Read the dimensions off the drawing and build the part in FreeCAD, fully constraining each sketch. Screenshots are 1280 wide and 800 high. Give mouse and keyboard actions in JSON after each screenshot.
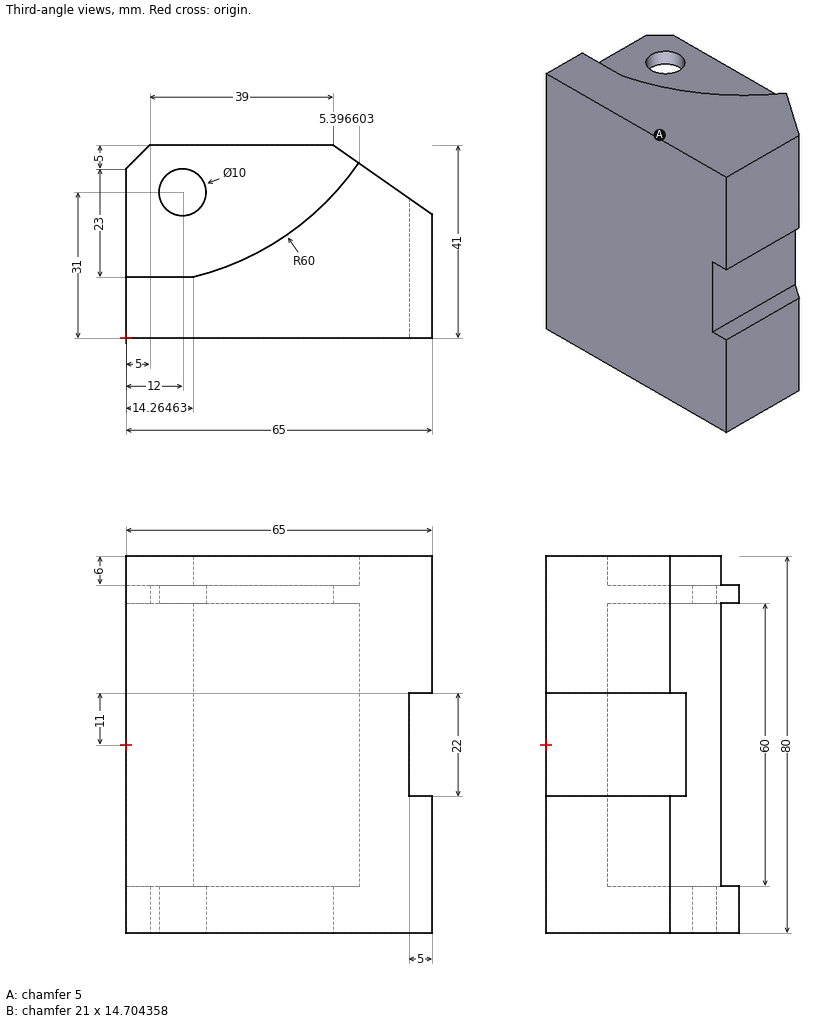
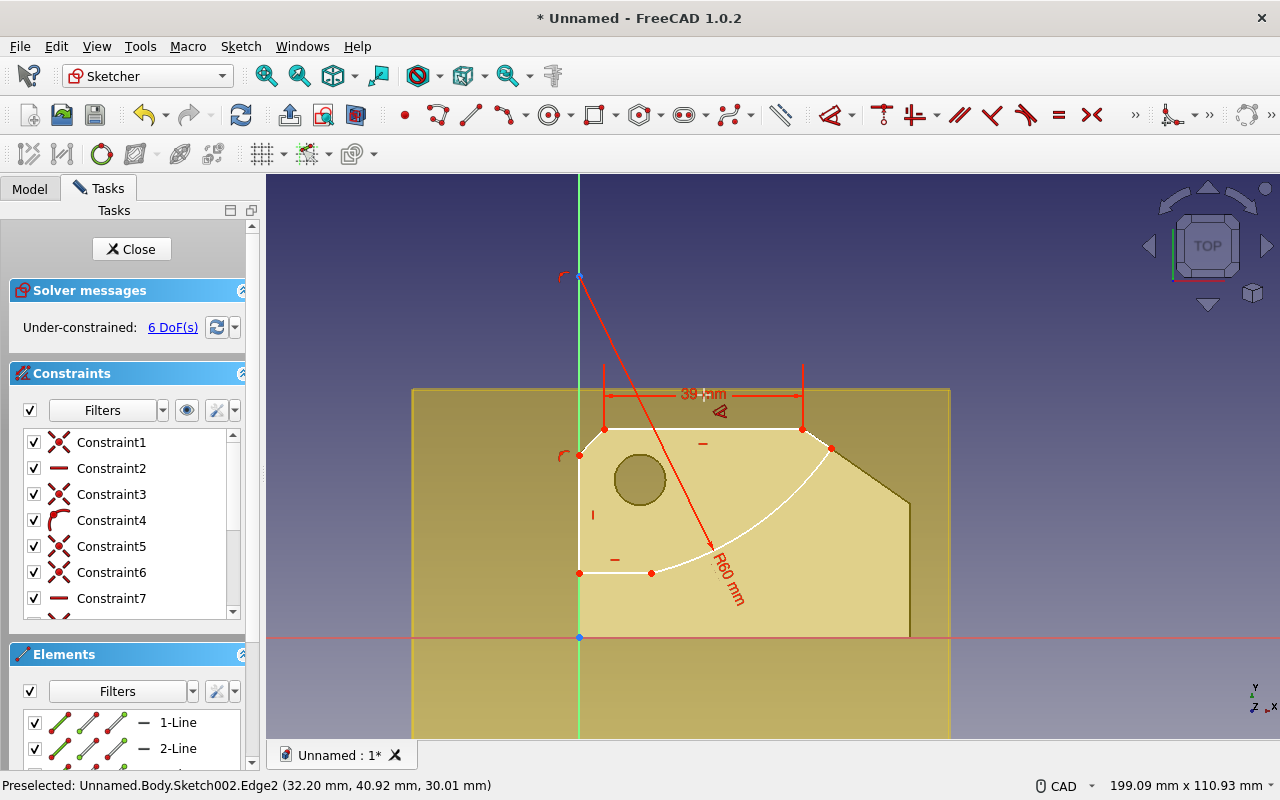
{"action": "left_click", "coordinate": [579, 491]}
{"action": "left_click", "coordinate": [545, 514]}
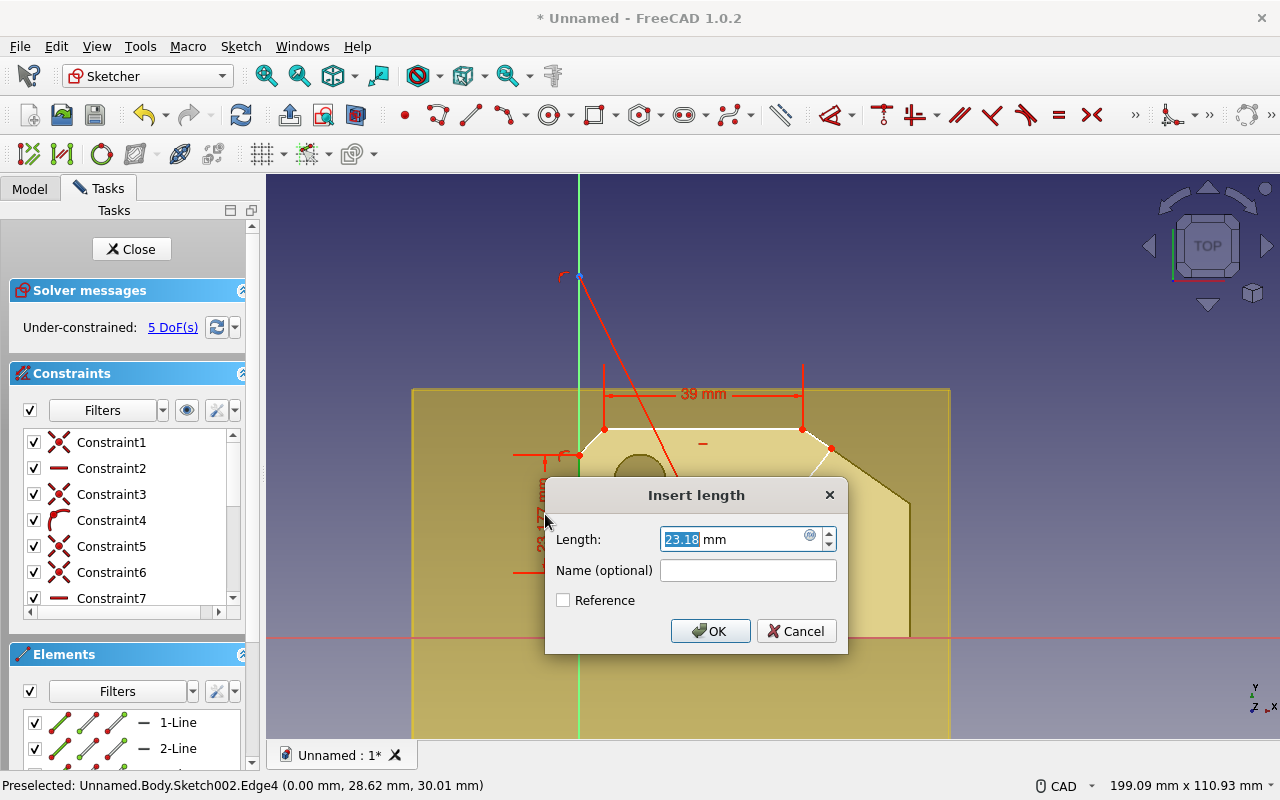
{"action": "type", "text": "23"}
{"action": "key", "text": "Return"}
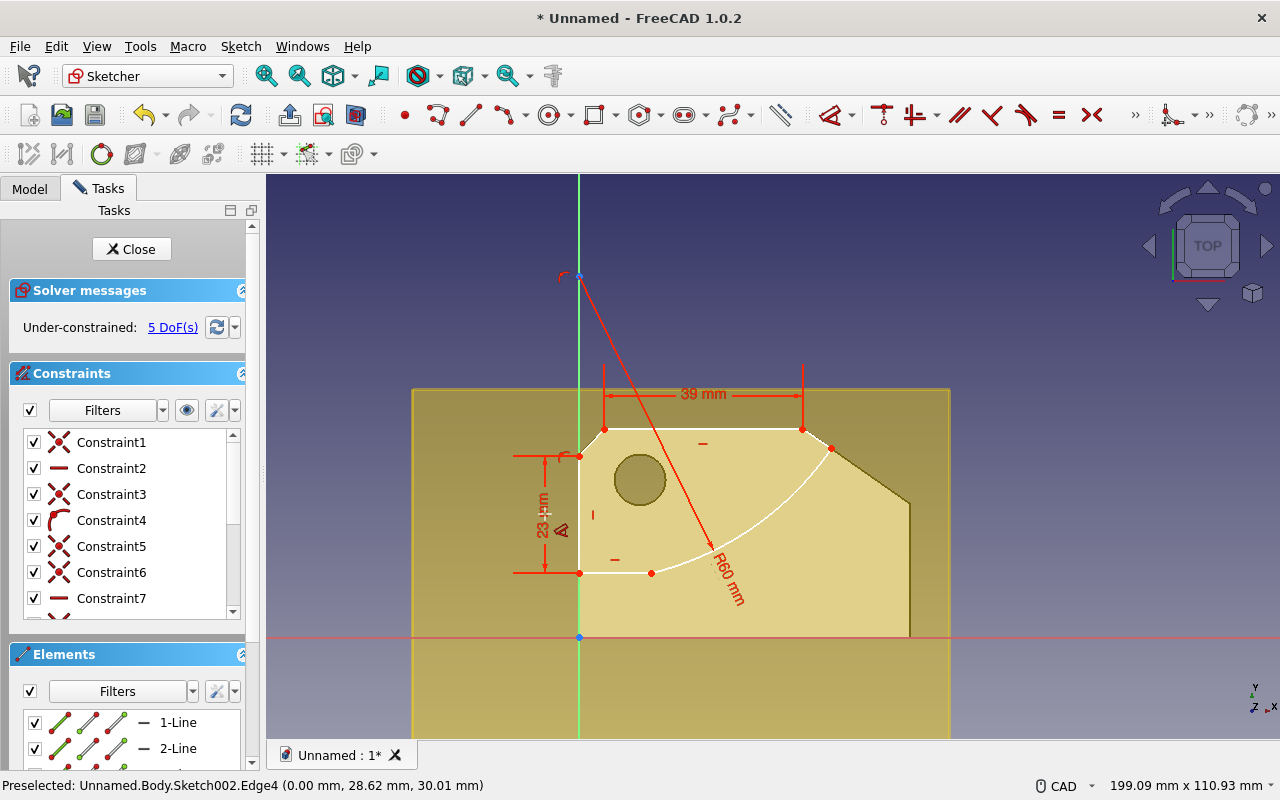
{"action": "scroll", "coordinate": [604, 429], "scroll_direction": "up", "scroll_amount": 3}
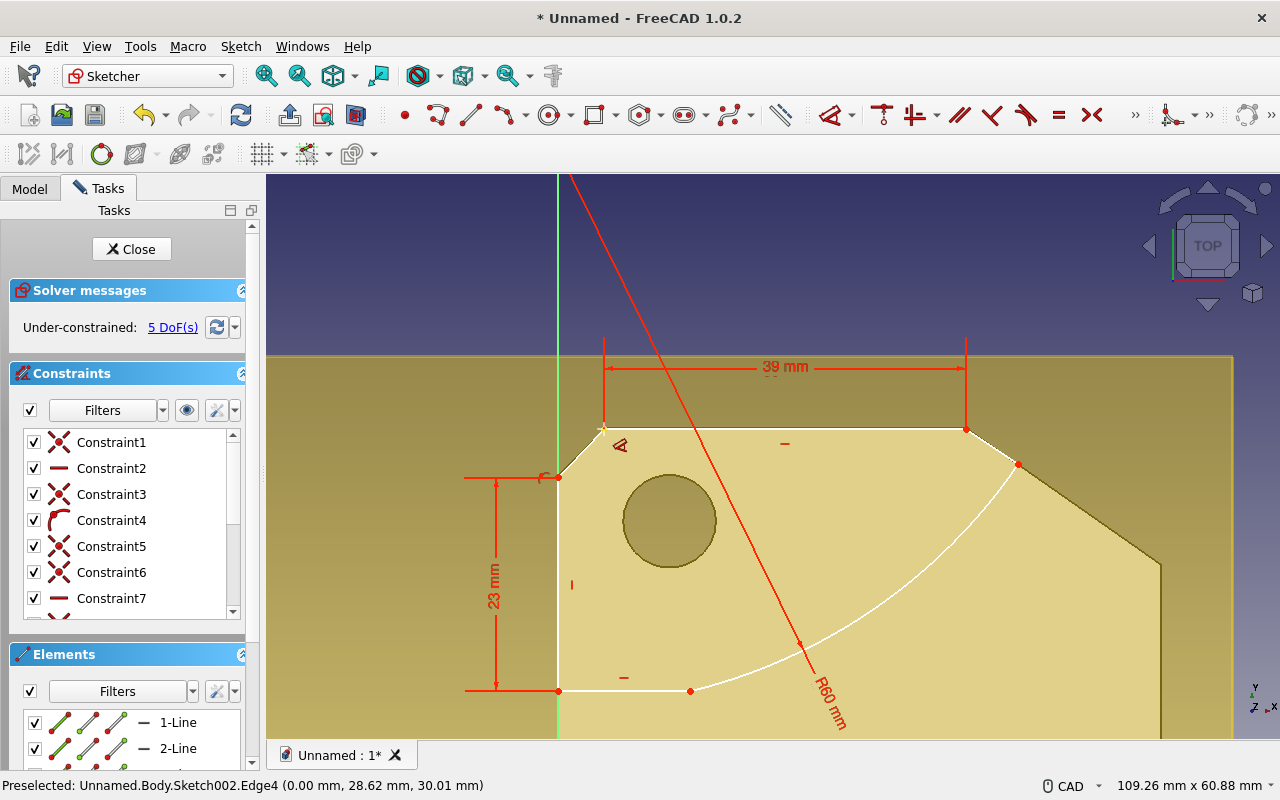
{"action": "left_click", "coordinate": [604, 429]}
{"action": "left_click", "coordinate": [581, 395]}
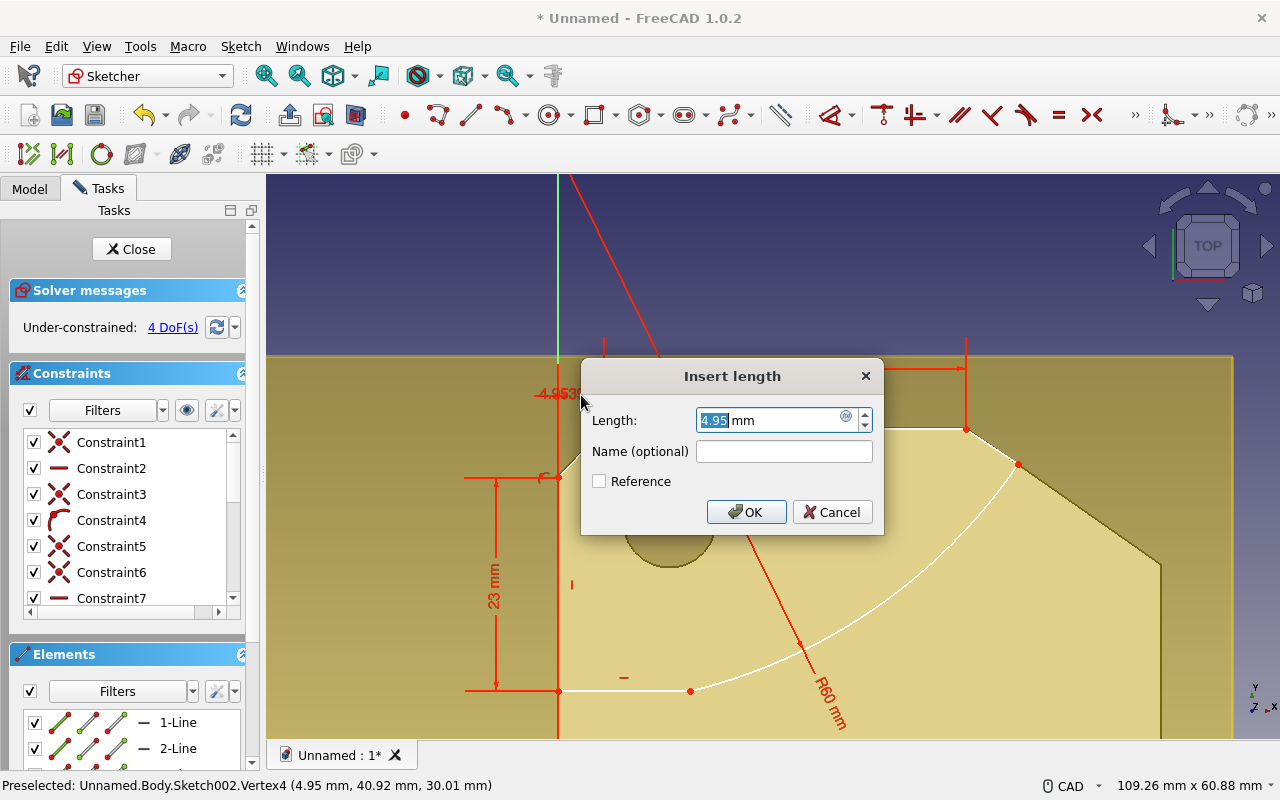
{"action": "type", "text": "5"}
{"action": "key", "text": "Return"}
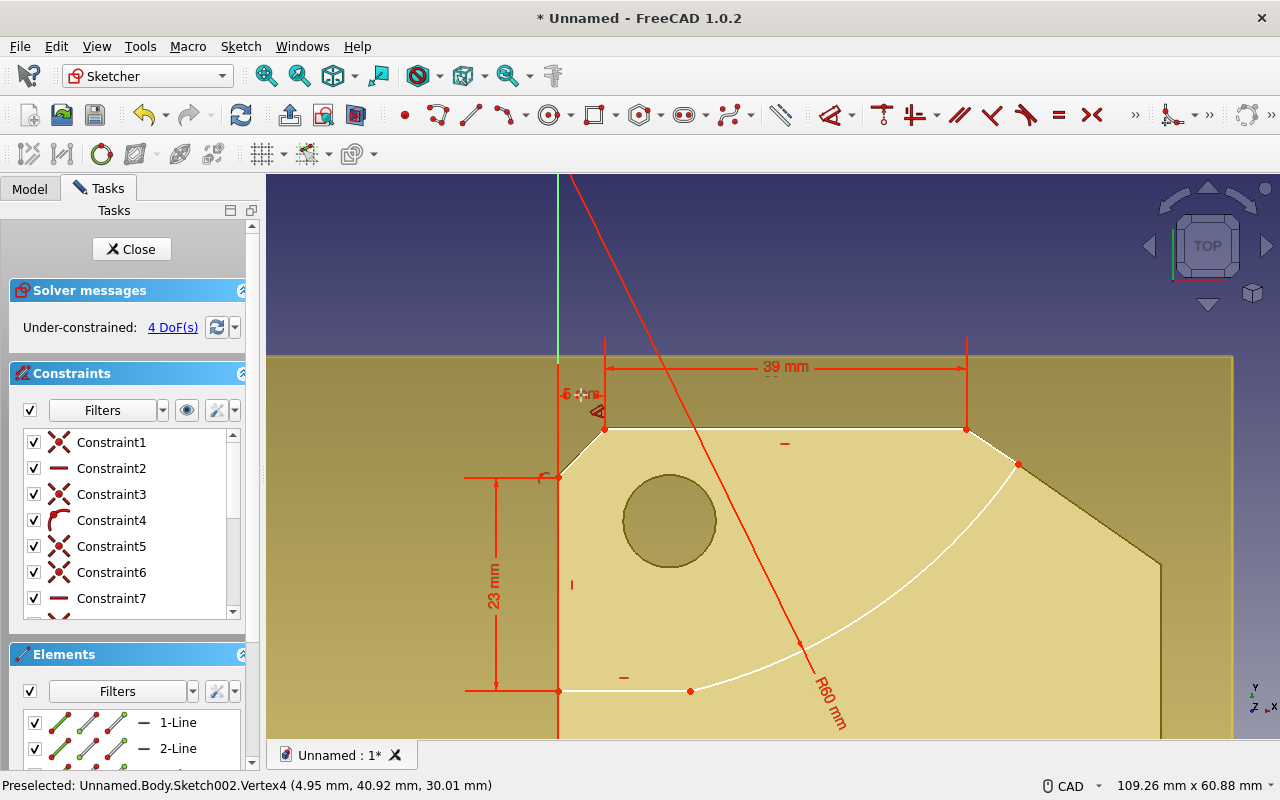
{"action": "left_click", "coordinate": [591, 444]}
{"action": "left_click", "coordinate": [524, 454]}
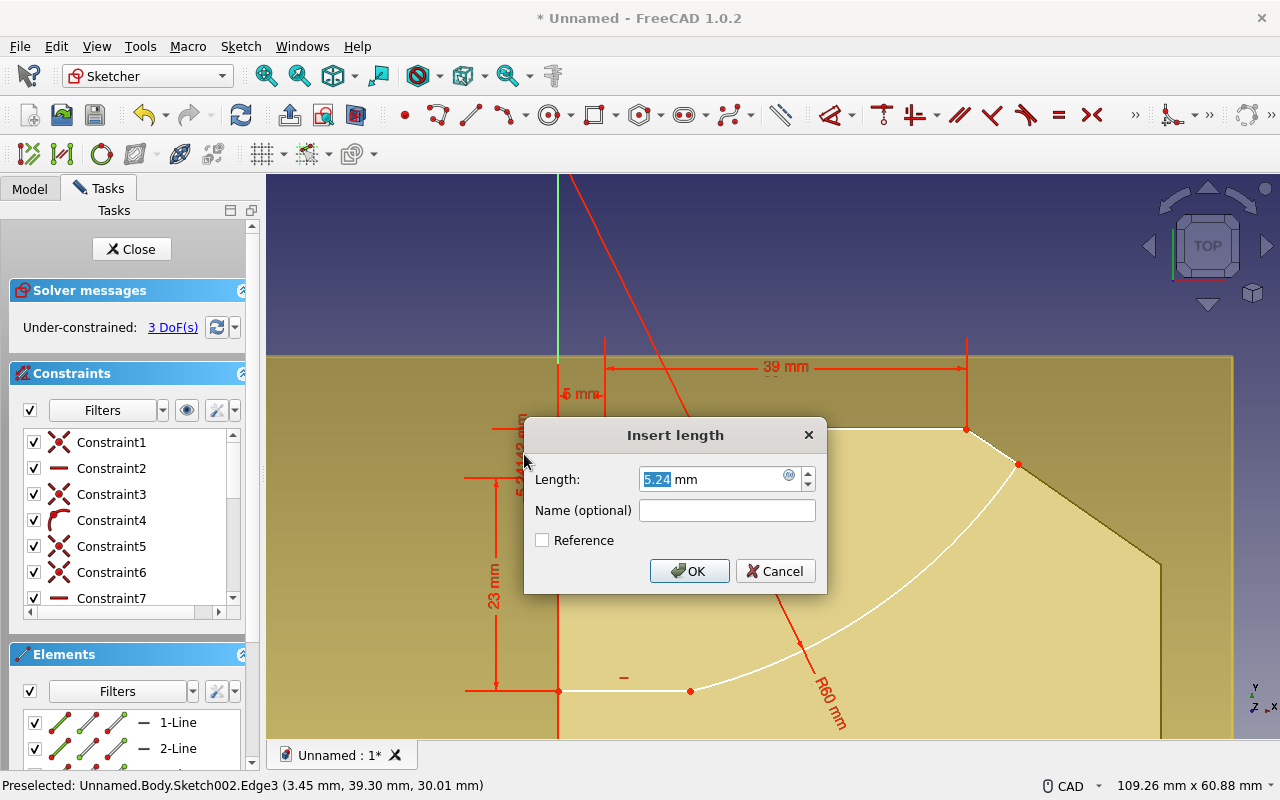
{"action": "type", "text": "5"}
{"action": "key", "text": "Return"}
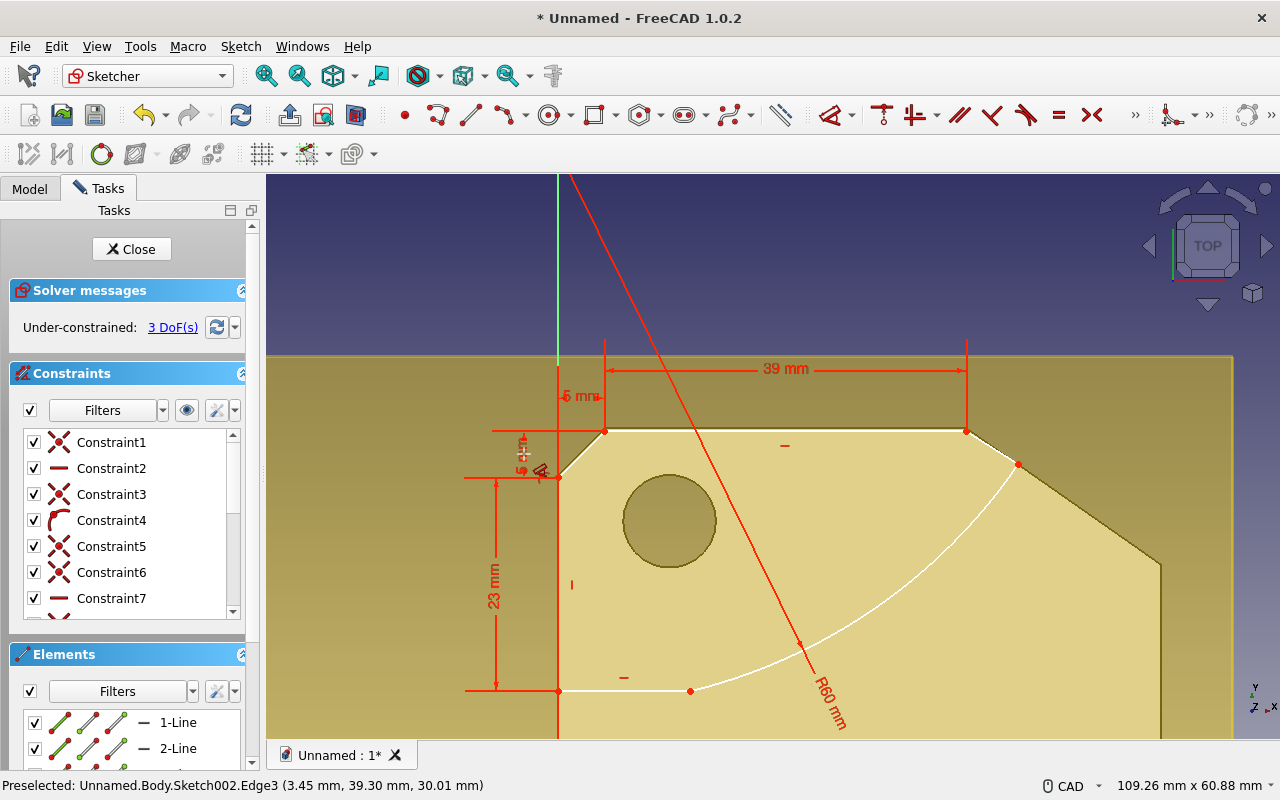
{"action": "left_click", "coordinate": [967, 431]}
{"action": "left_click", "coordinate": [524, 507]}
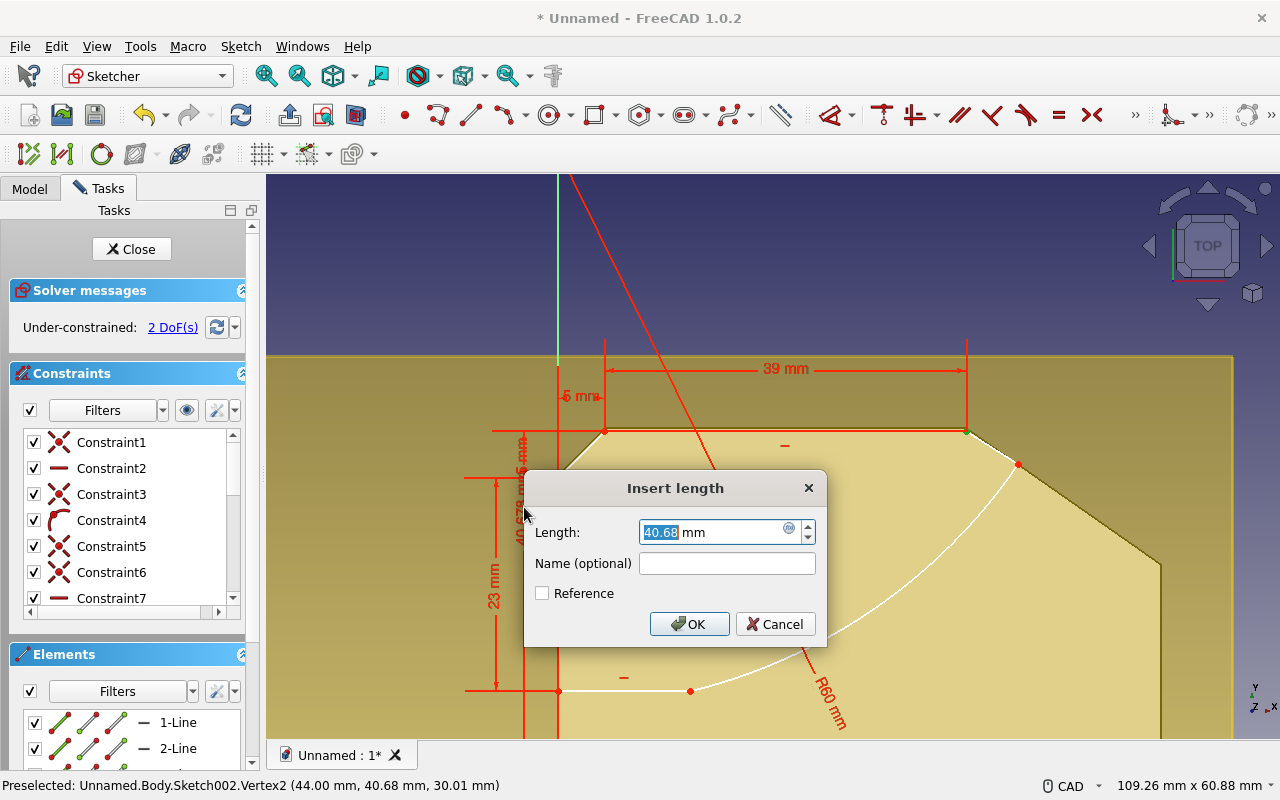
{"action": "type", "text": "41"}
{"action": "key", "text": "Return"}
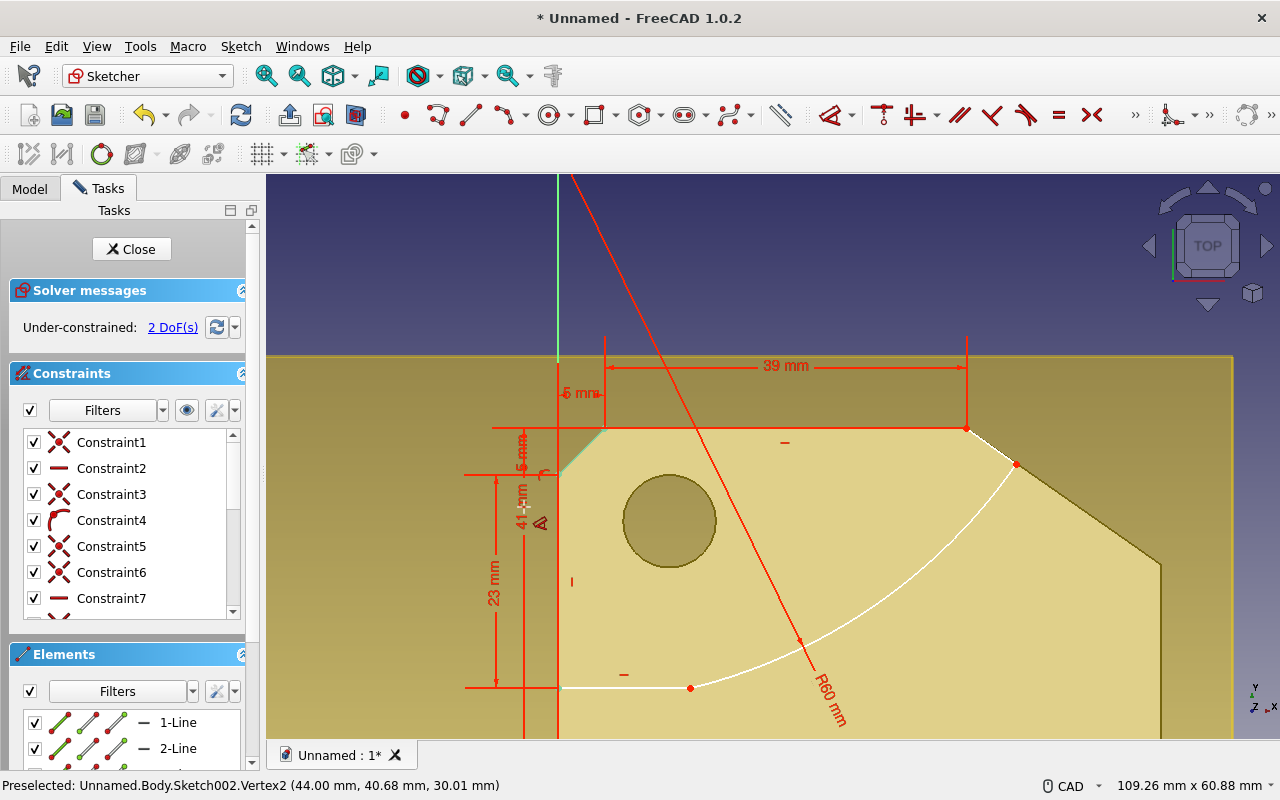
{"action": "left_click", "coordinate": [598, 688]}
{"action": "left_click", "coordinate": [624, 654]}